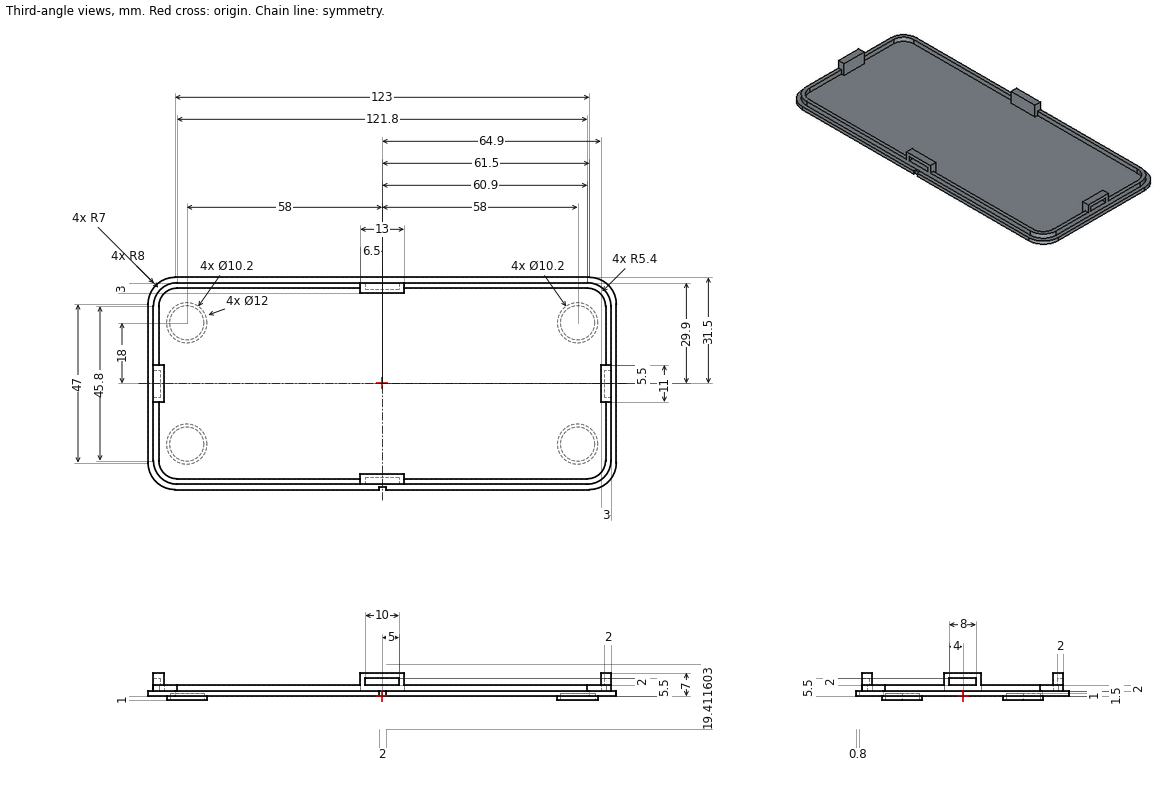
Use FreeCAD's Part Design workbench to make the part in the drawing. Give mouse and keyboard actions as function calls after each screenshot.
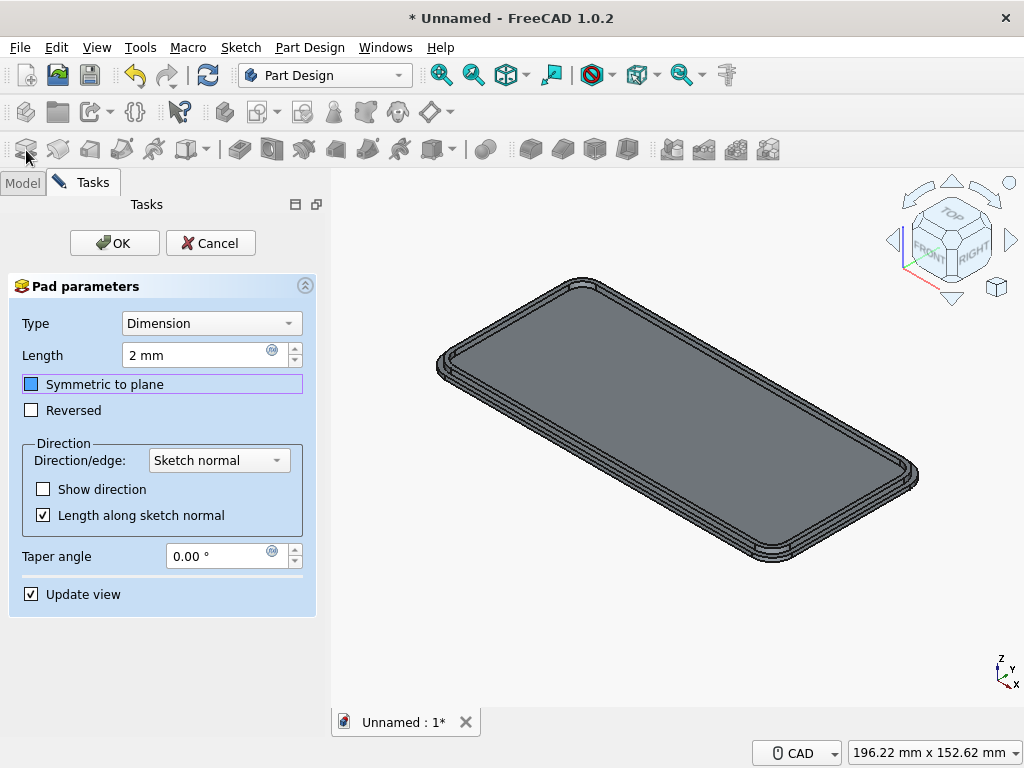
click(115, 243)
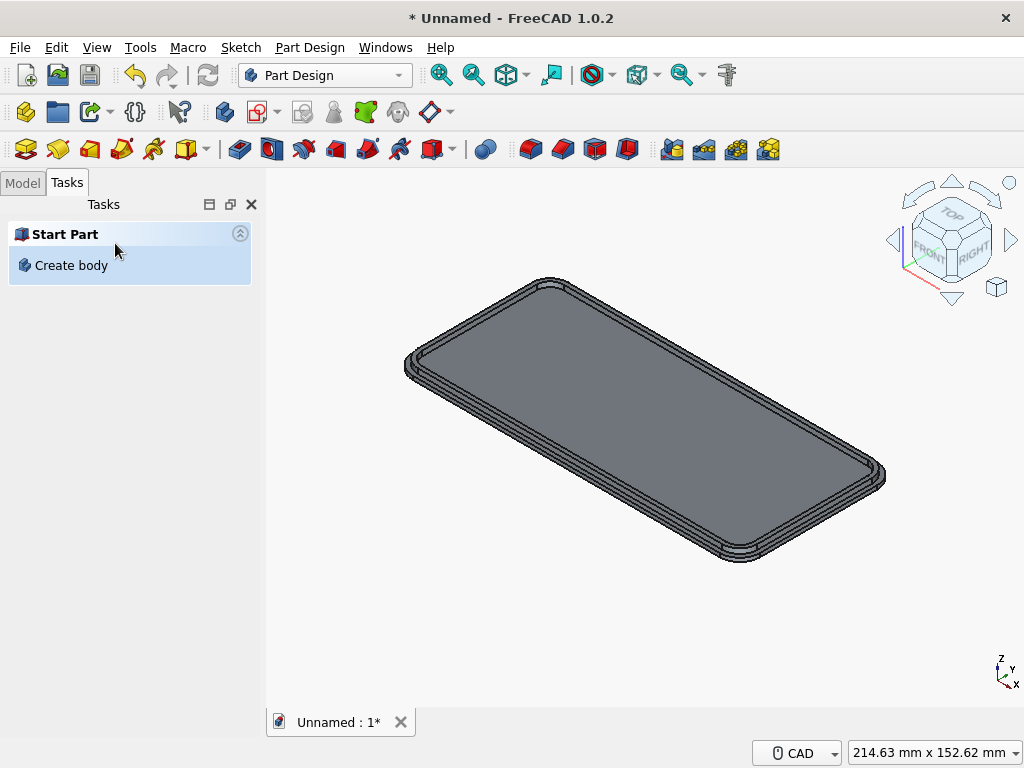
scroll(535, 281, up, 10)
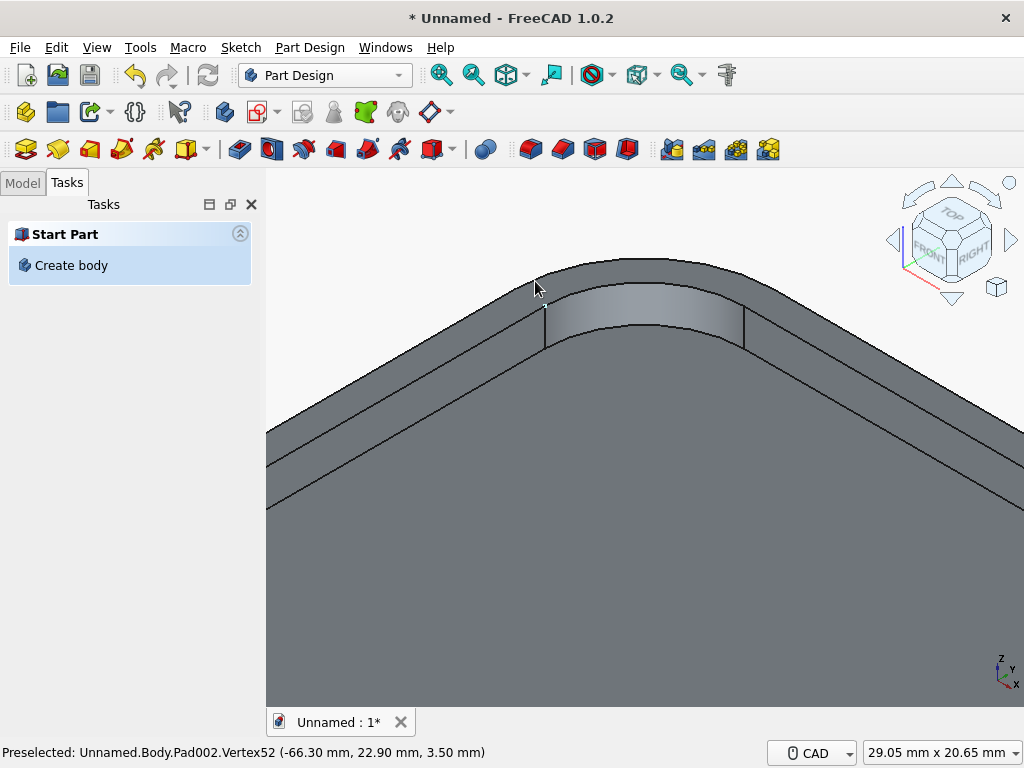
click(533, 289)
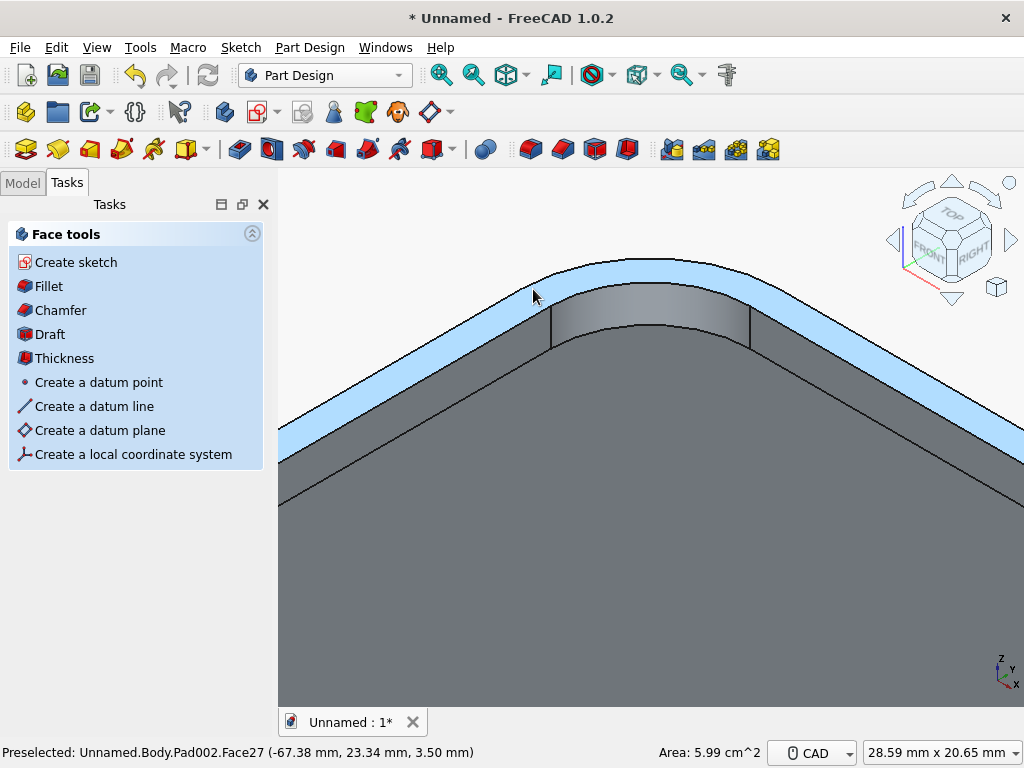
click(258, 112)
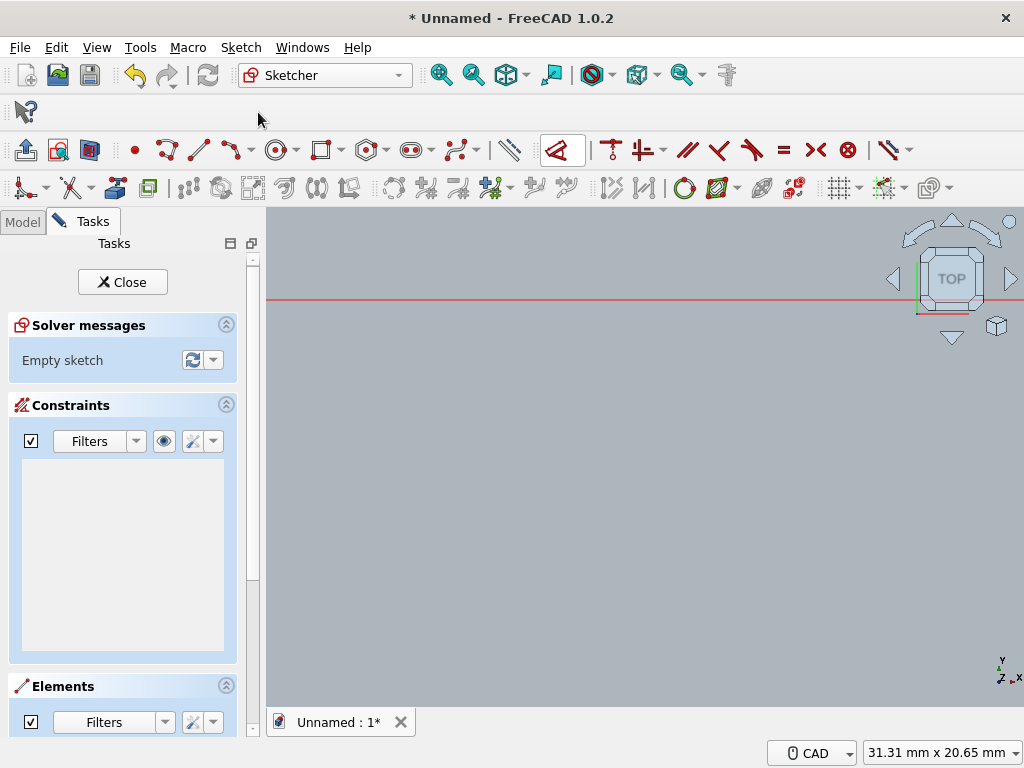
scroll(473, 477, down, 11)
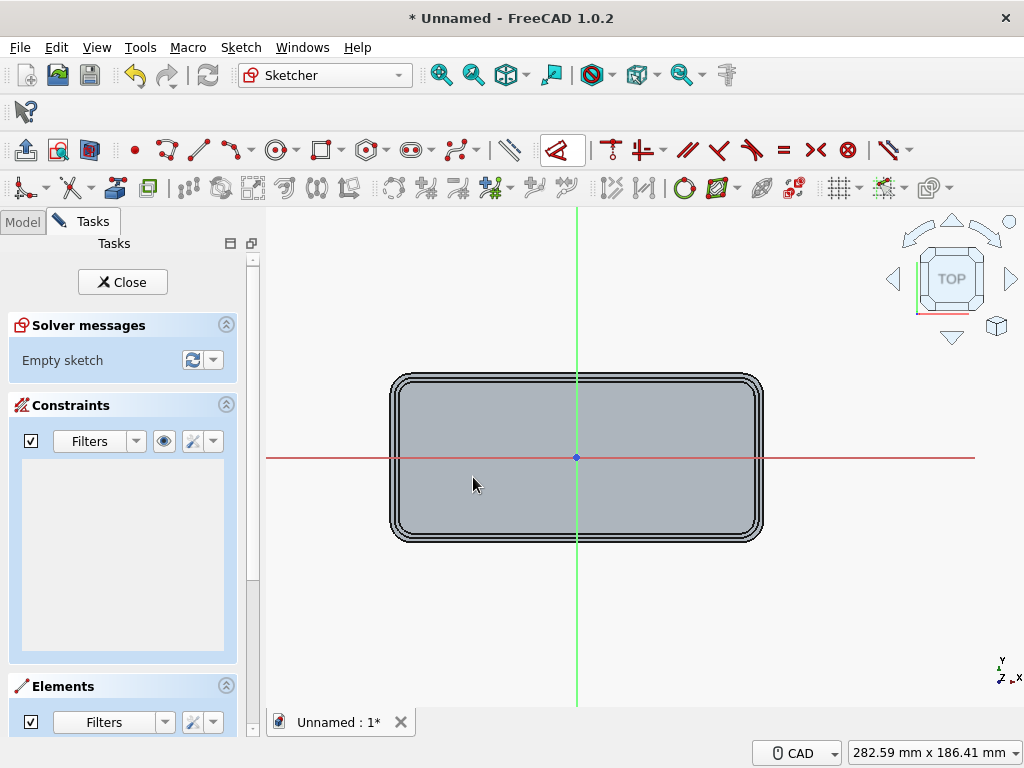
key(g)
key(r)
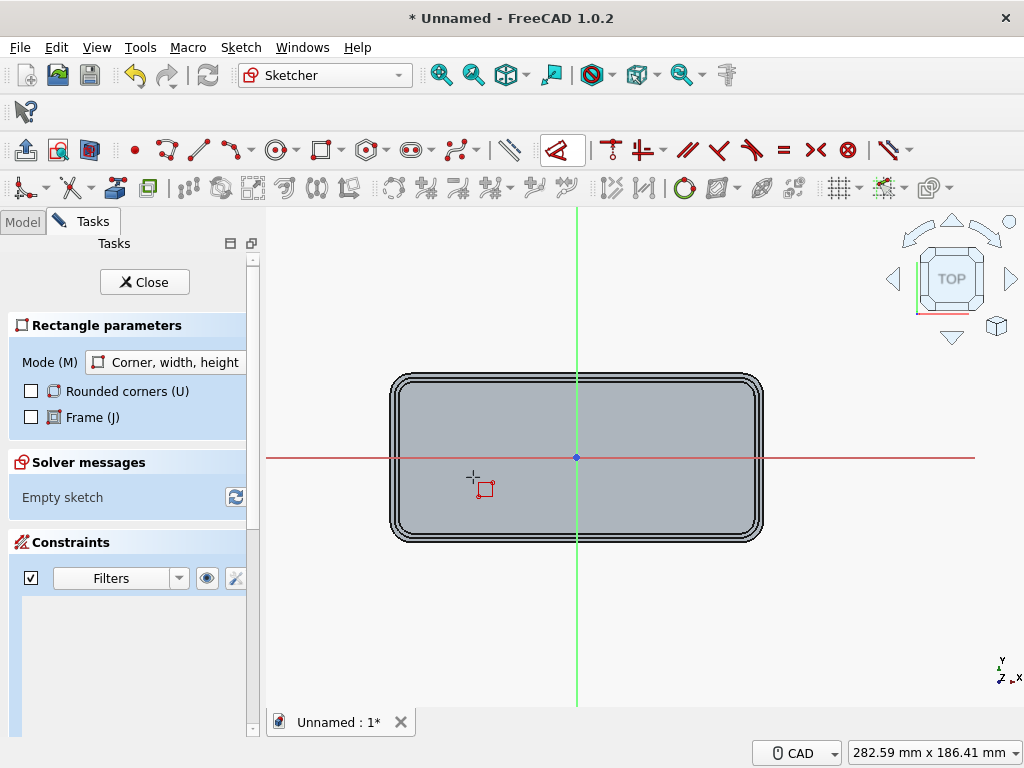
scroll(559, 378, up, 4)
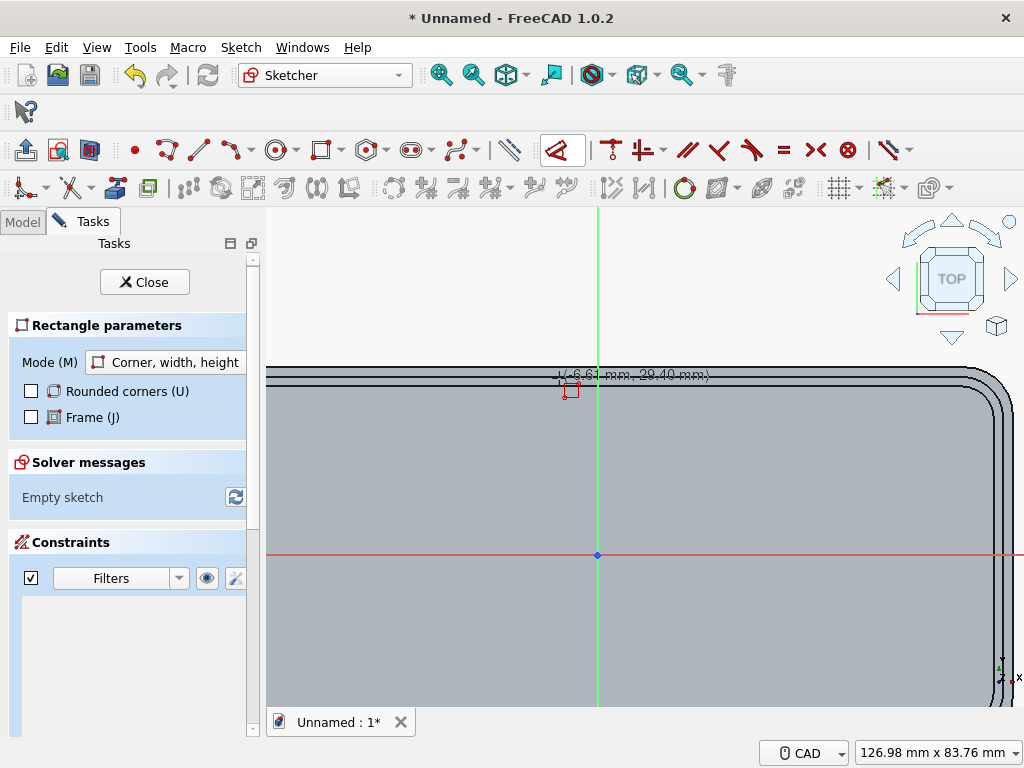
click(559, 377)
click(637, 395)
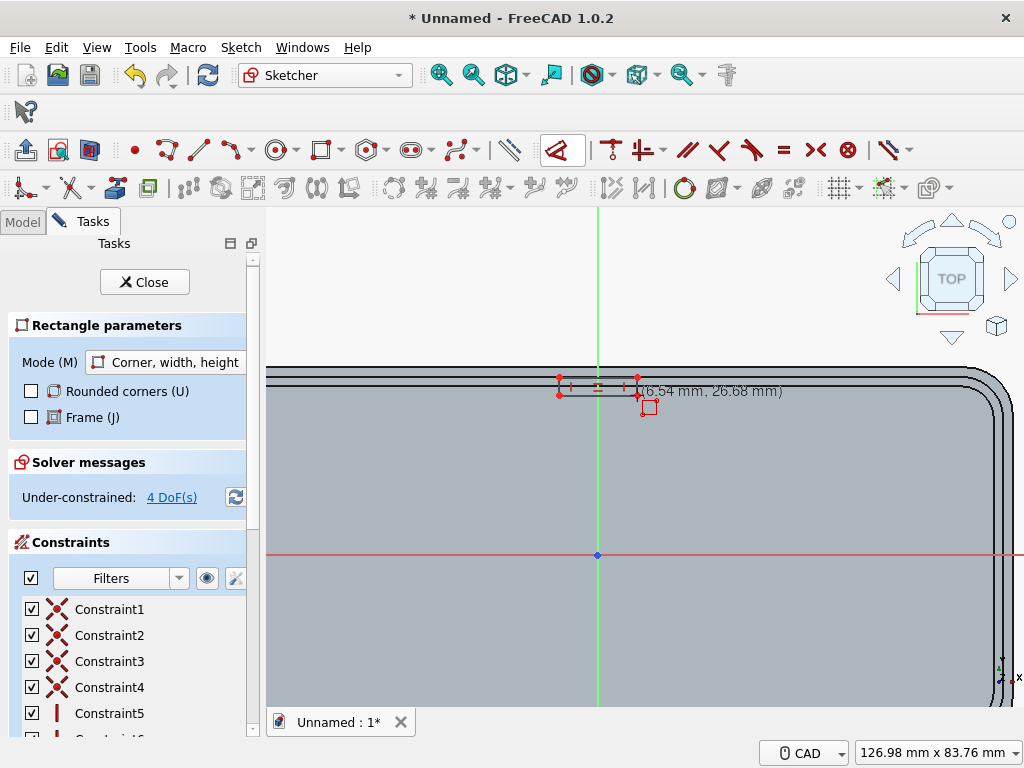
scroll(559, 377, down, 4)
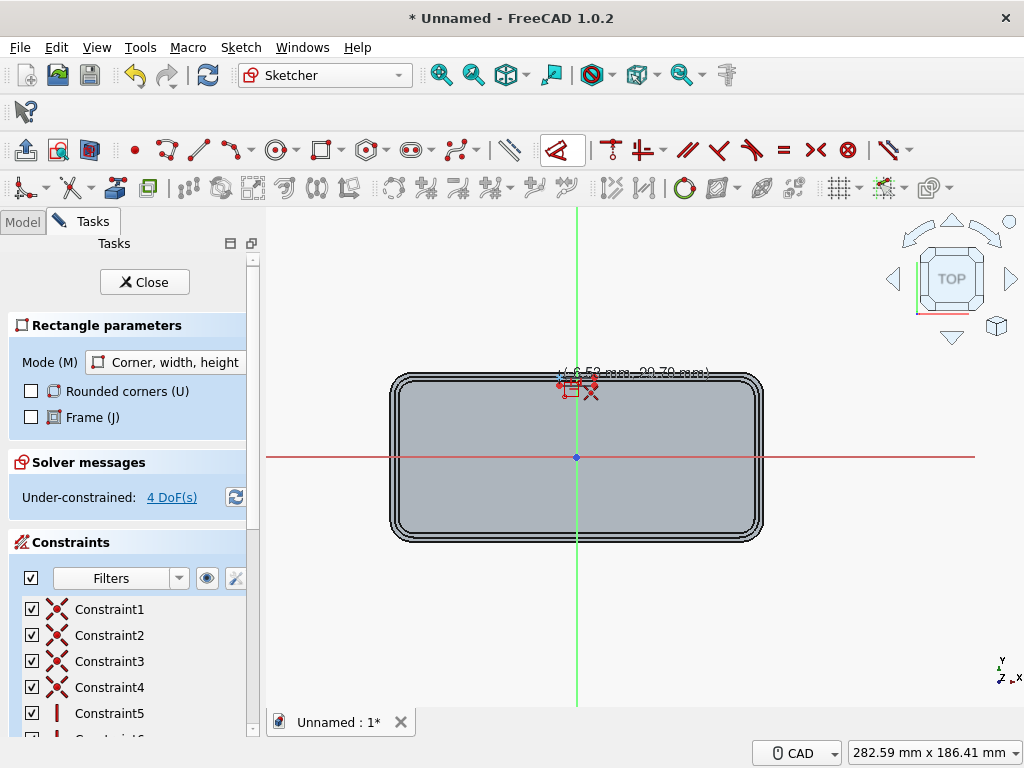
scroll(559, 529, up, 4)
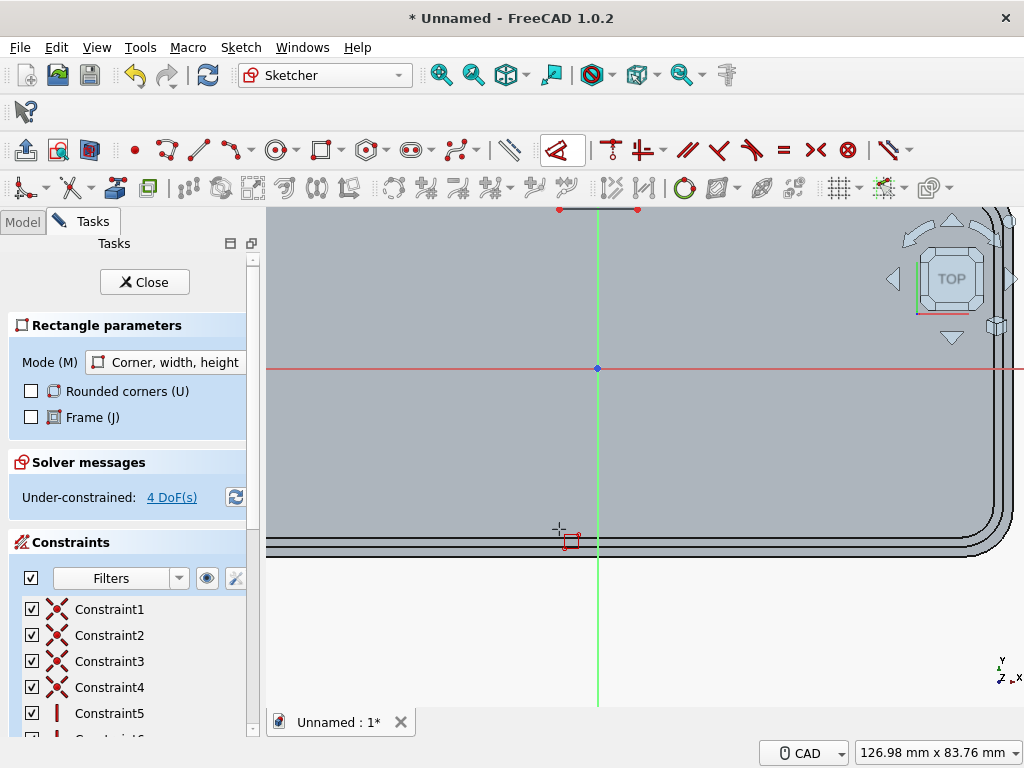
click(559, 529)
click(637, 547)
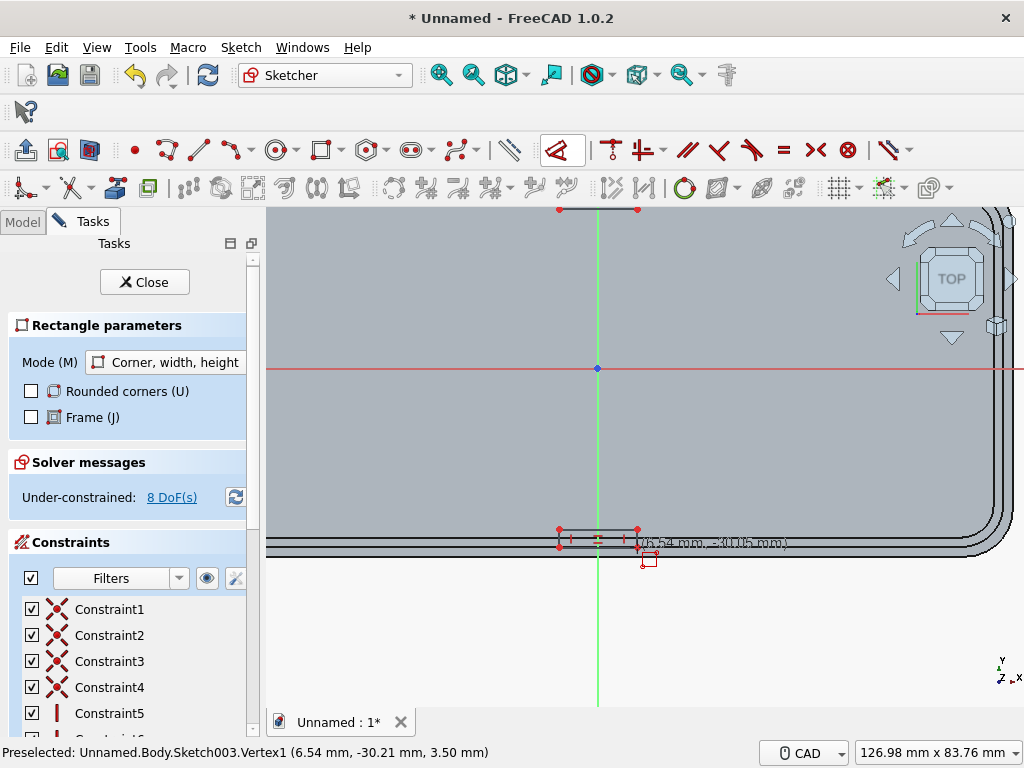
scroll(559, 529, down, 4)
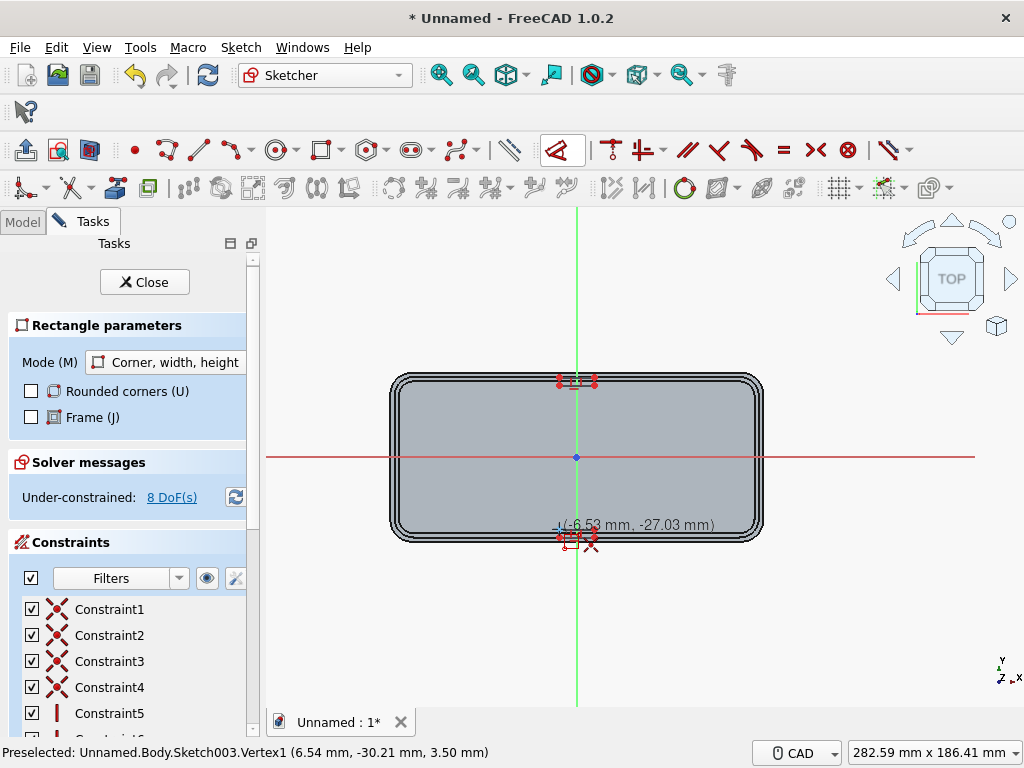
scroll(751, 443, up, 4)